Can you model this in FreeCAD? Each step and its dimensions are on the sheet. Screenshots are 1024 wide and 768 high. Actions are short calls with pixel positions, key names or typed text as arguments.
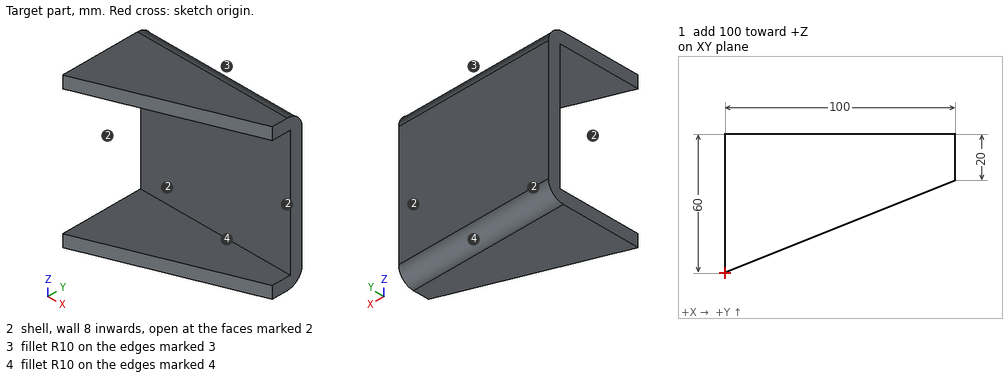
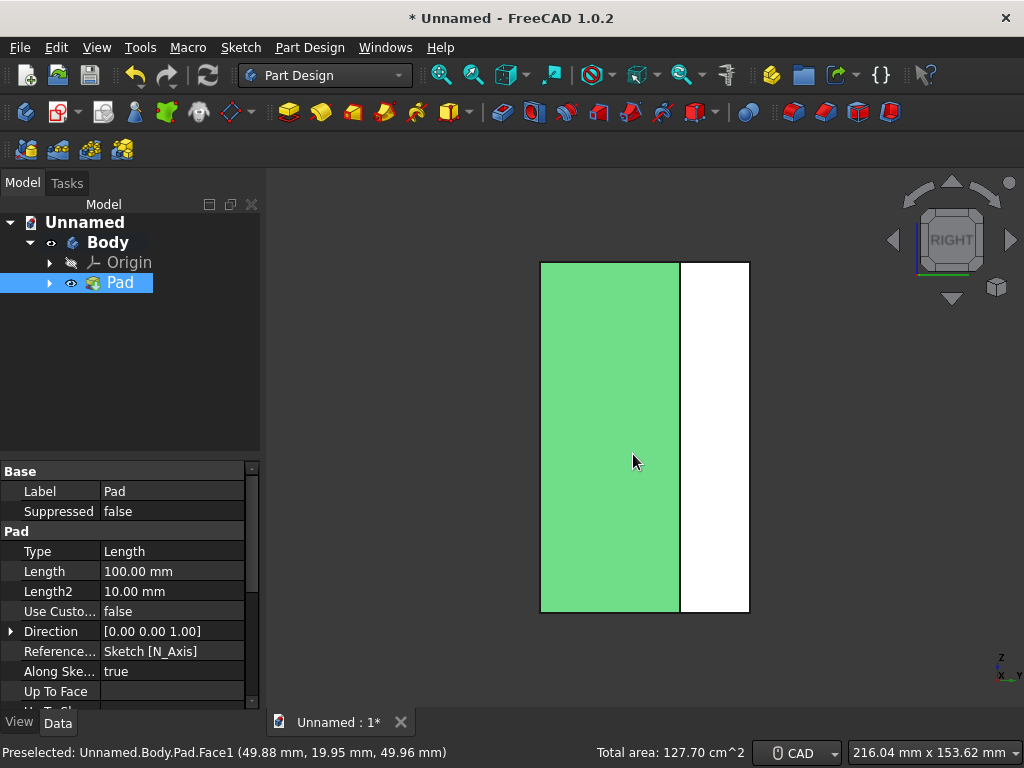
key(5)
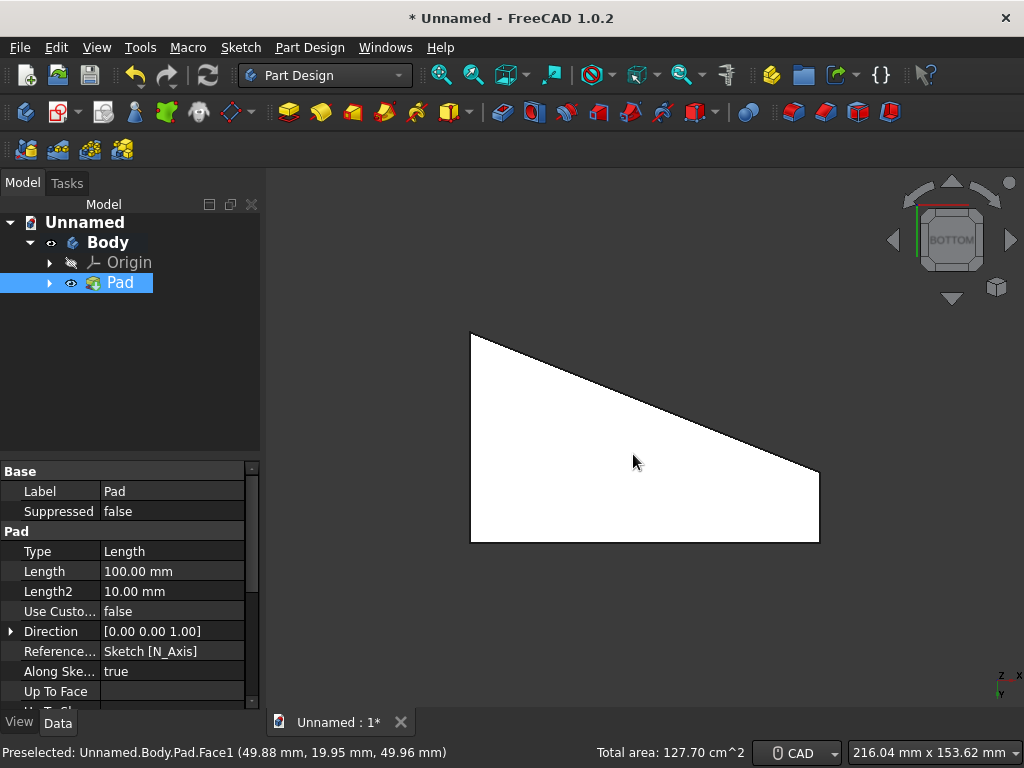
key(4)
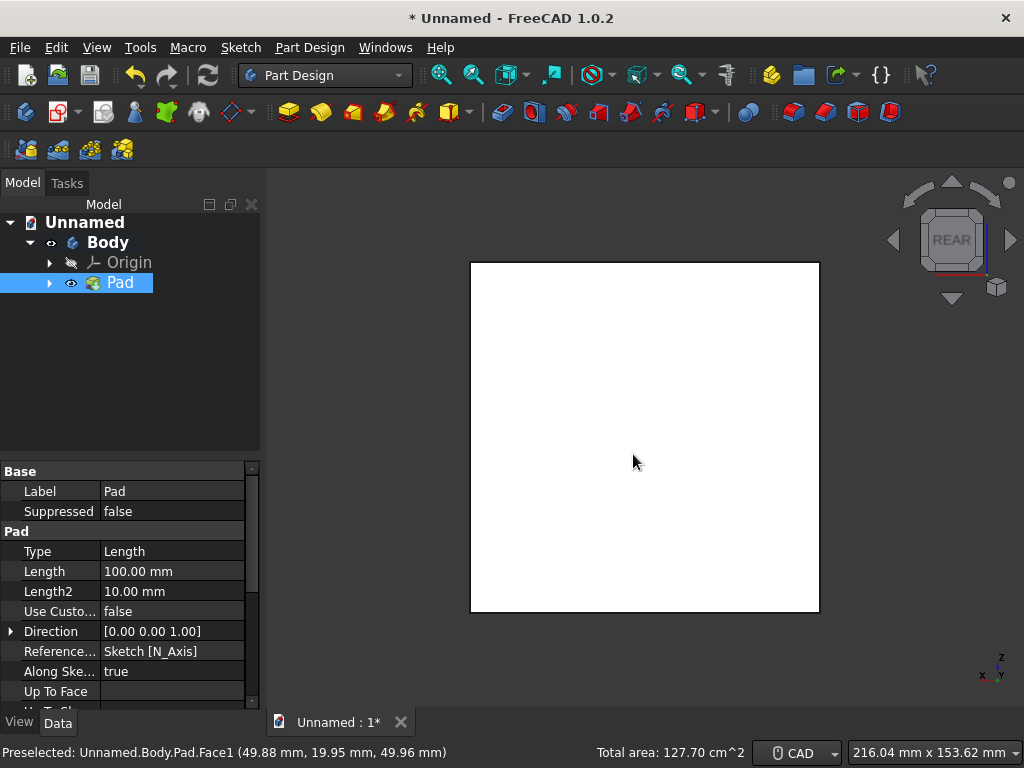
key(6)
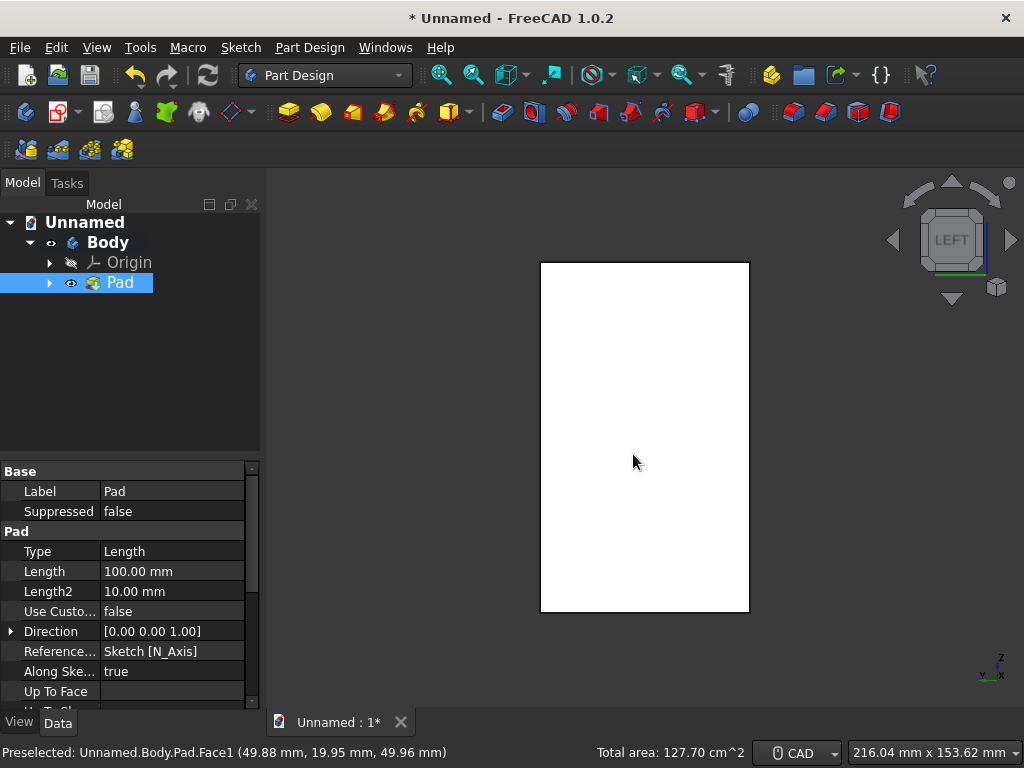
click(645, 386, ctrl)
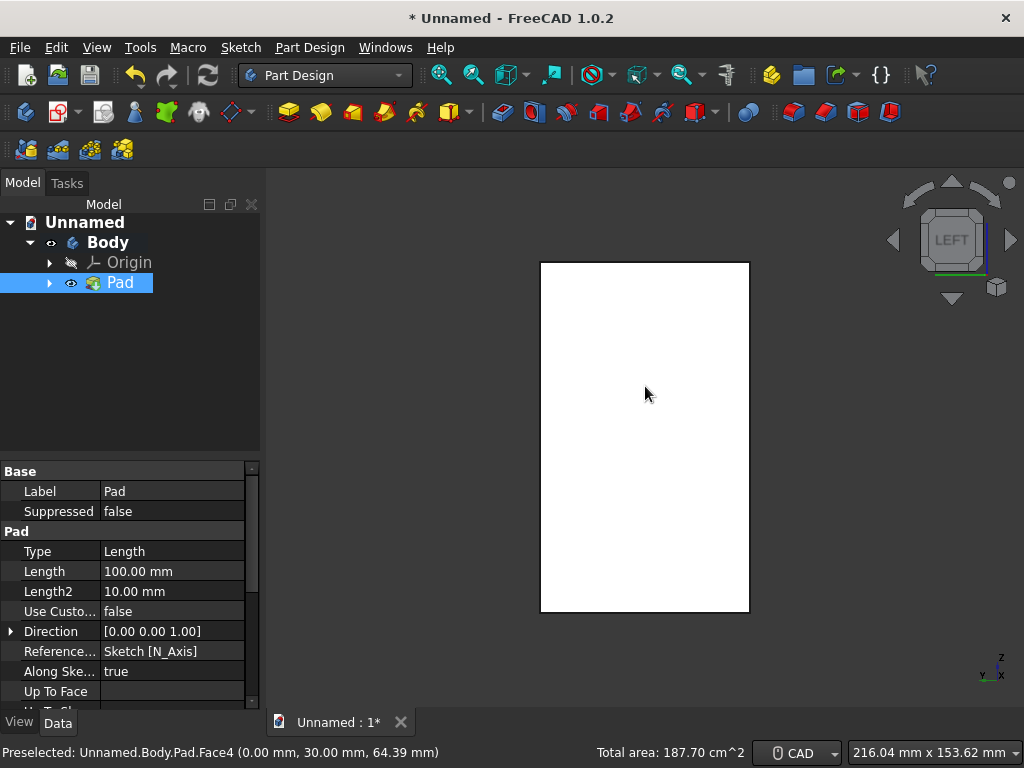
click(890, 112)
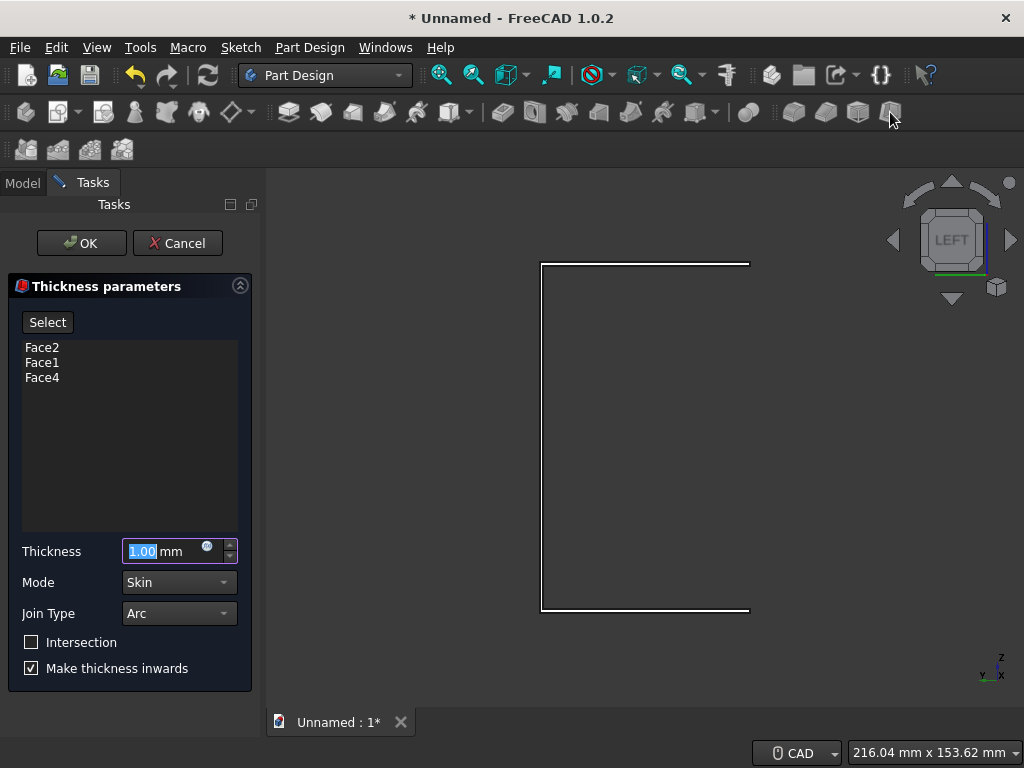
text(8)
key(Tab)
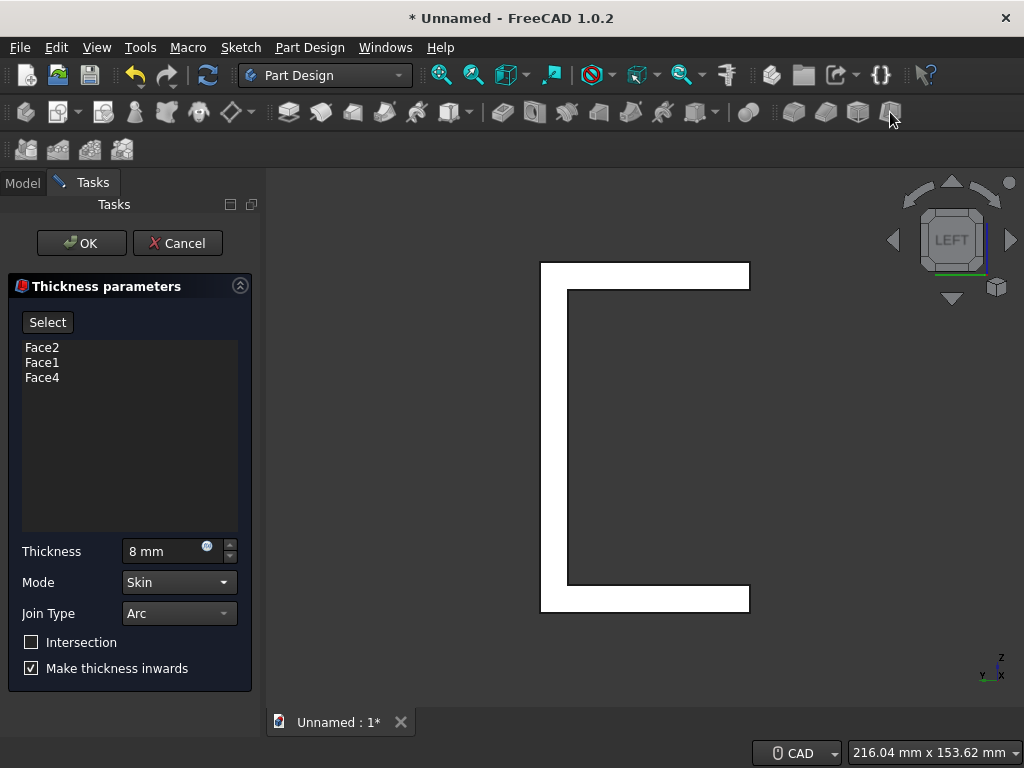
click(180, 614)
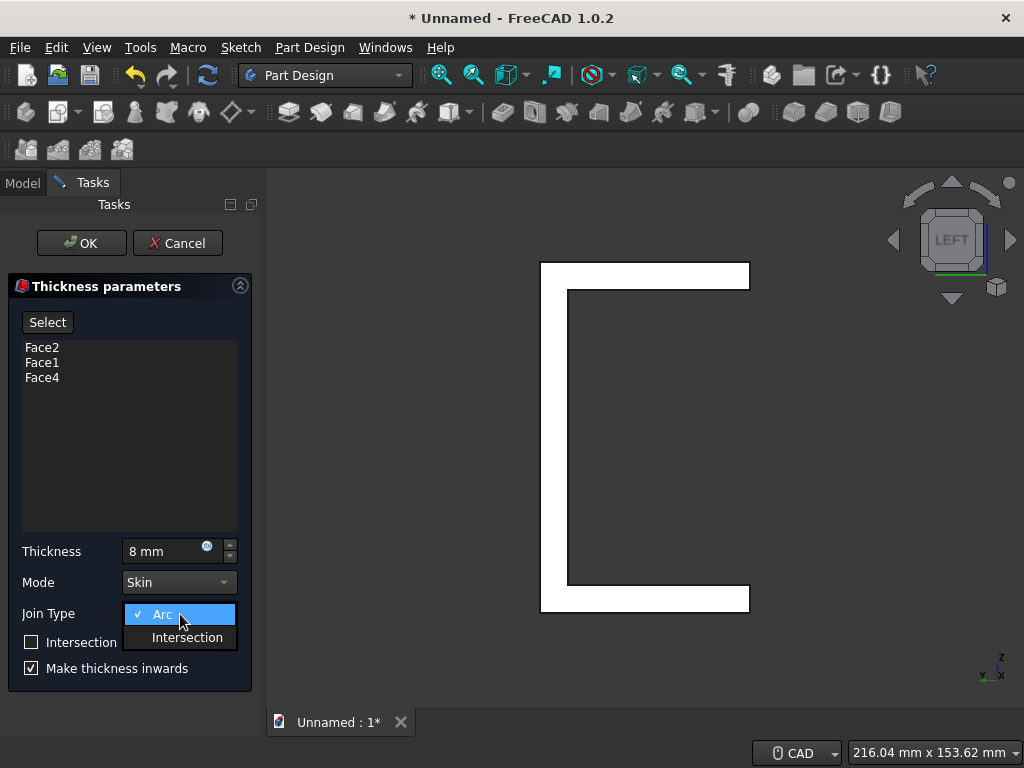
click(179, 638)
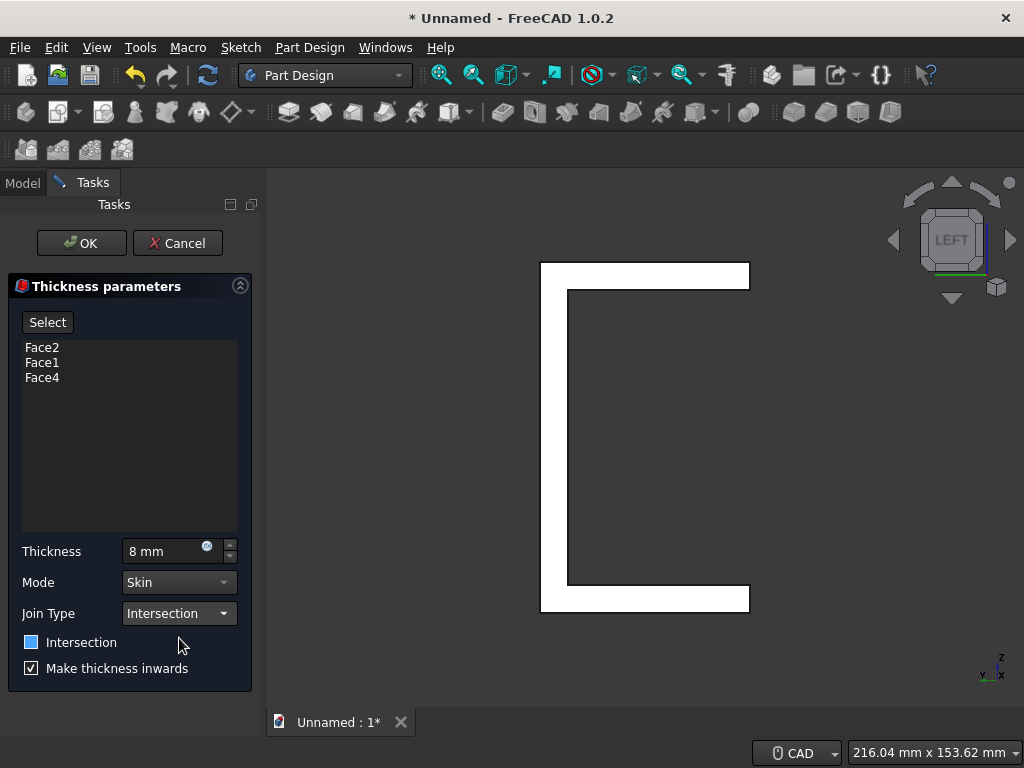
click(82, 243)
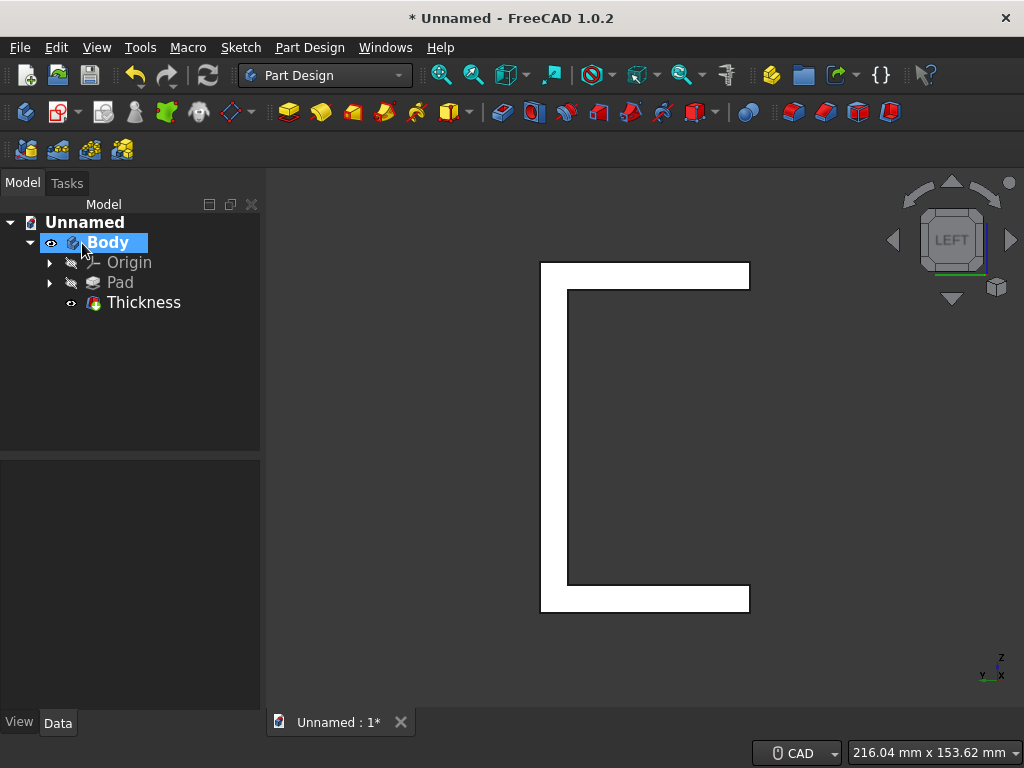
key(0)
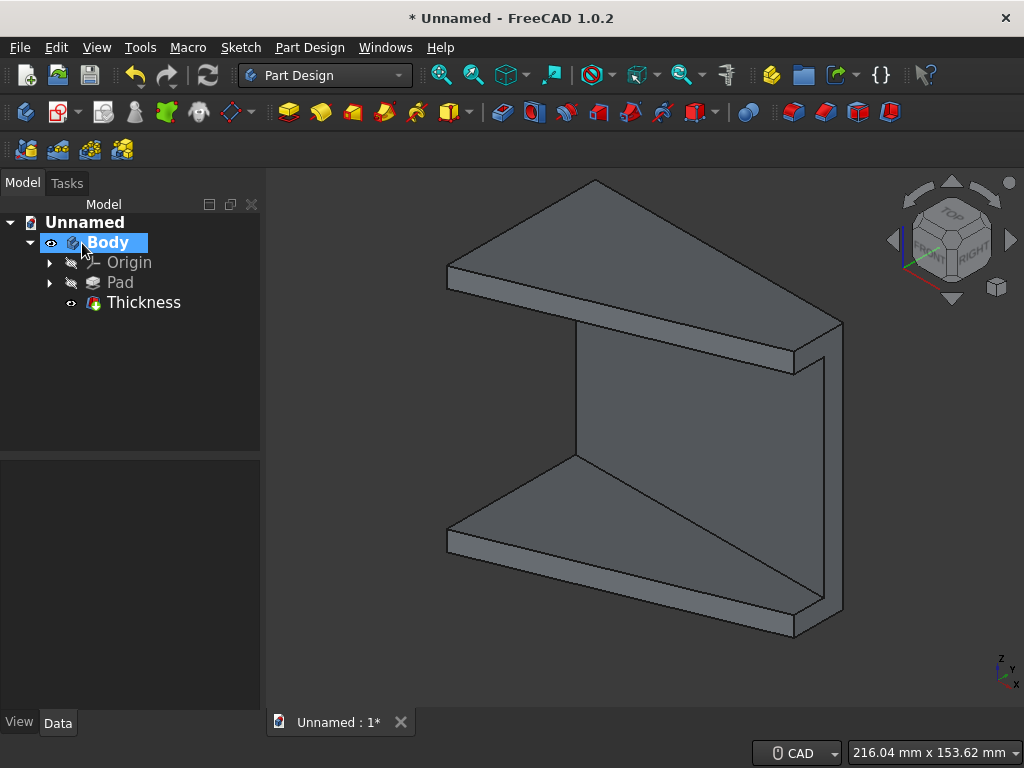
key(2)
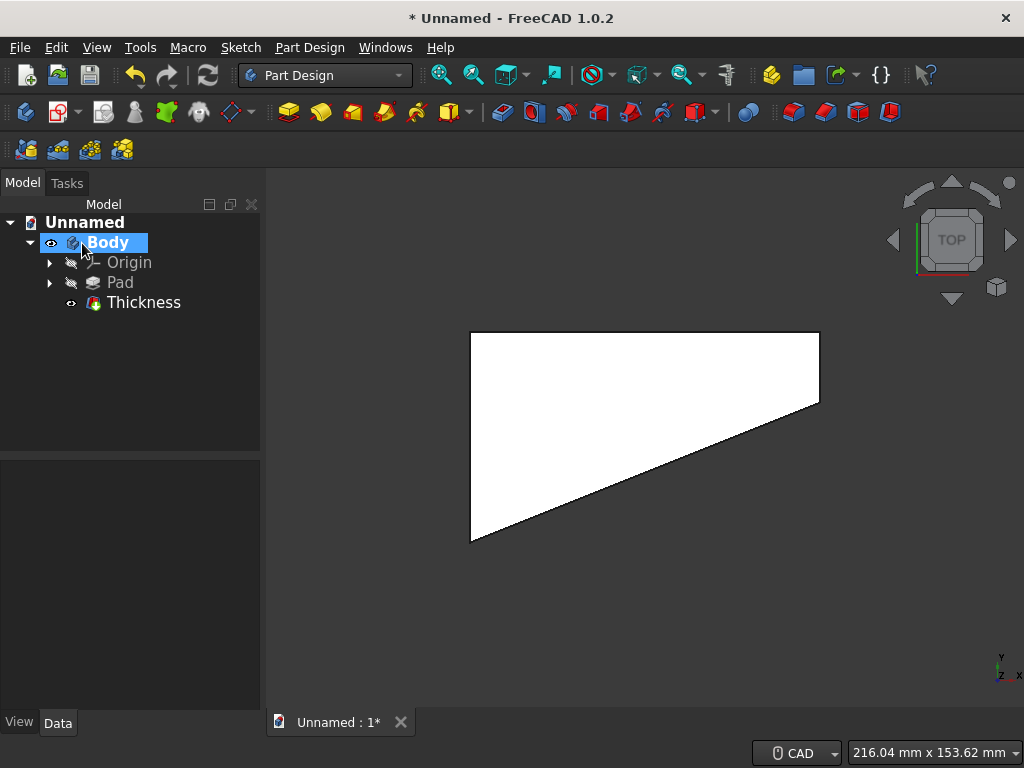
click(645, 331)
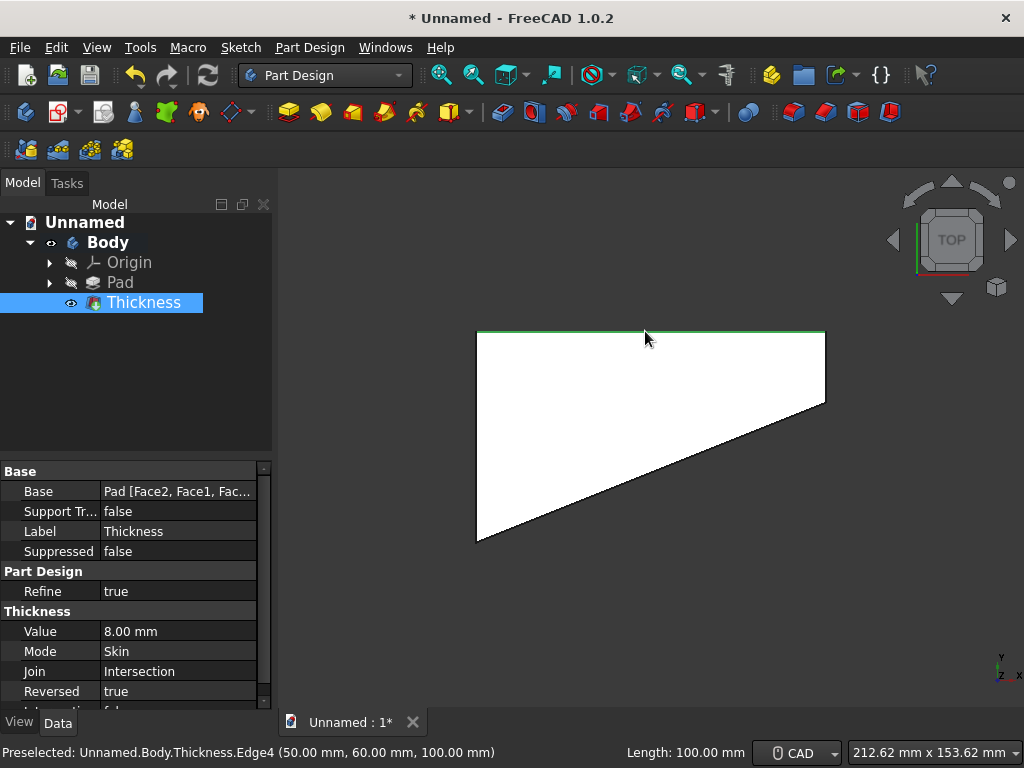
click(794, 112)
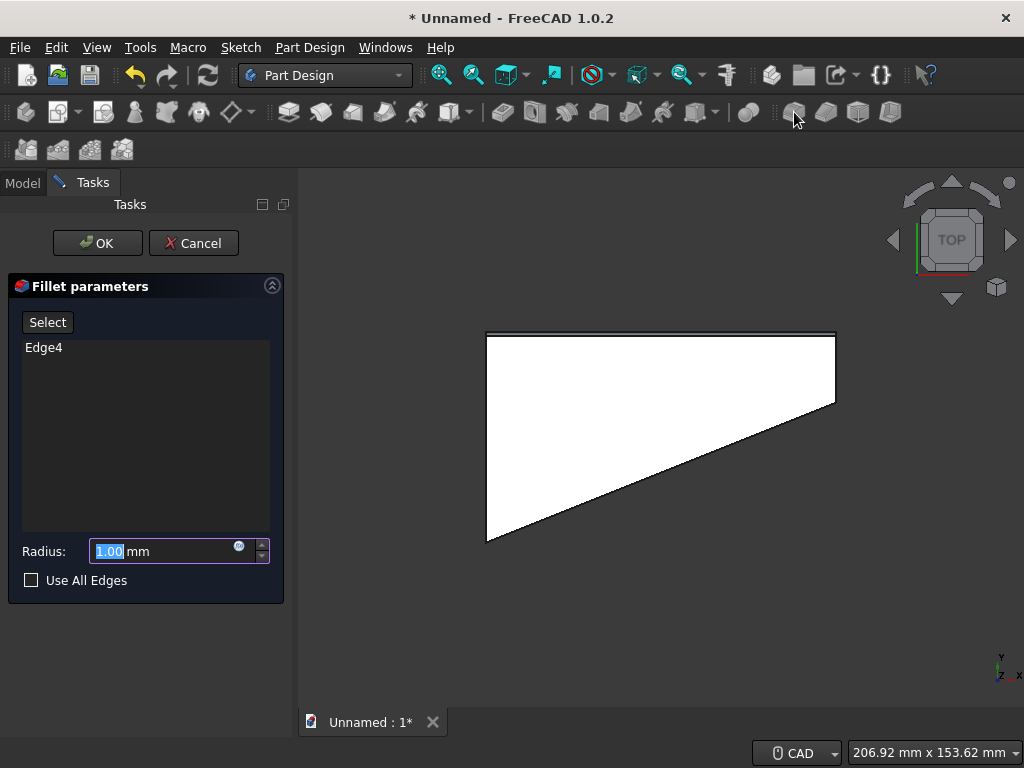
text(10)
key(Tab)